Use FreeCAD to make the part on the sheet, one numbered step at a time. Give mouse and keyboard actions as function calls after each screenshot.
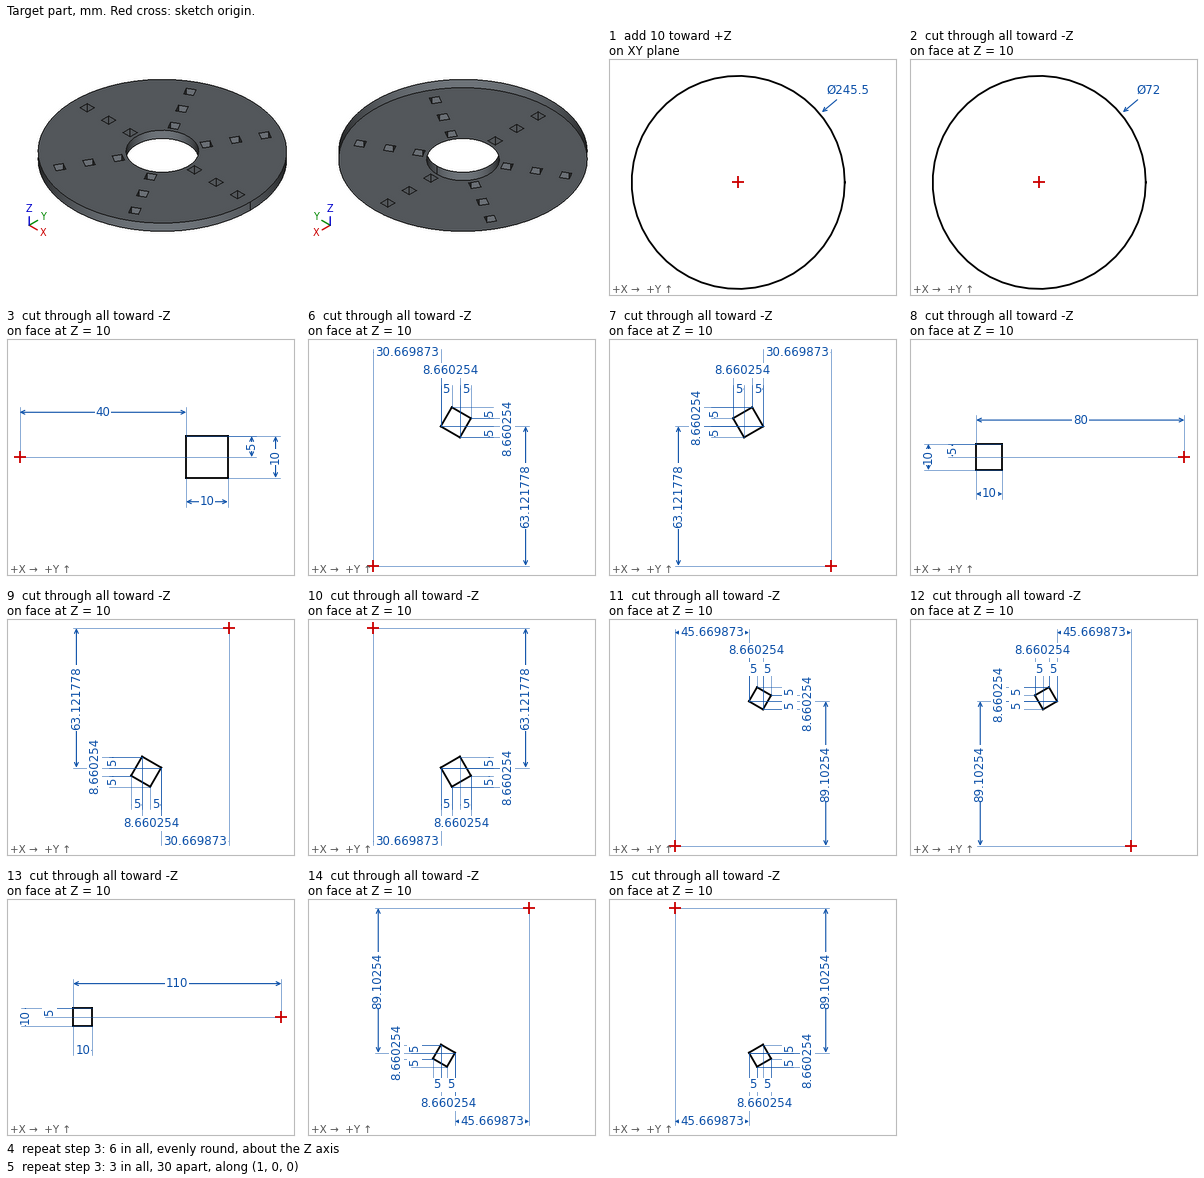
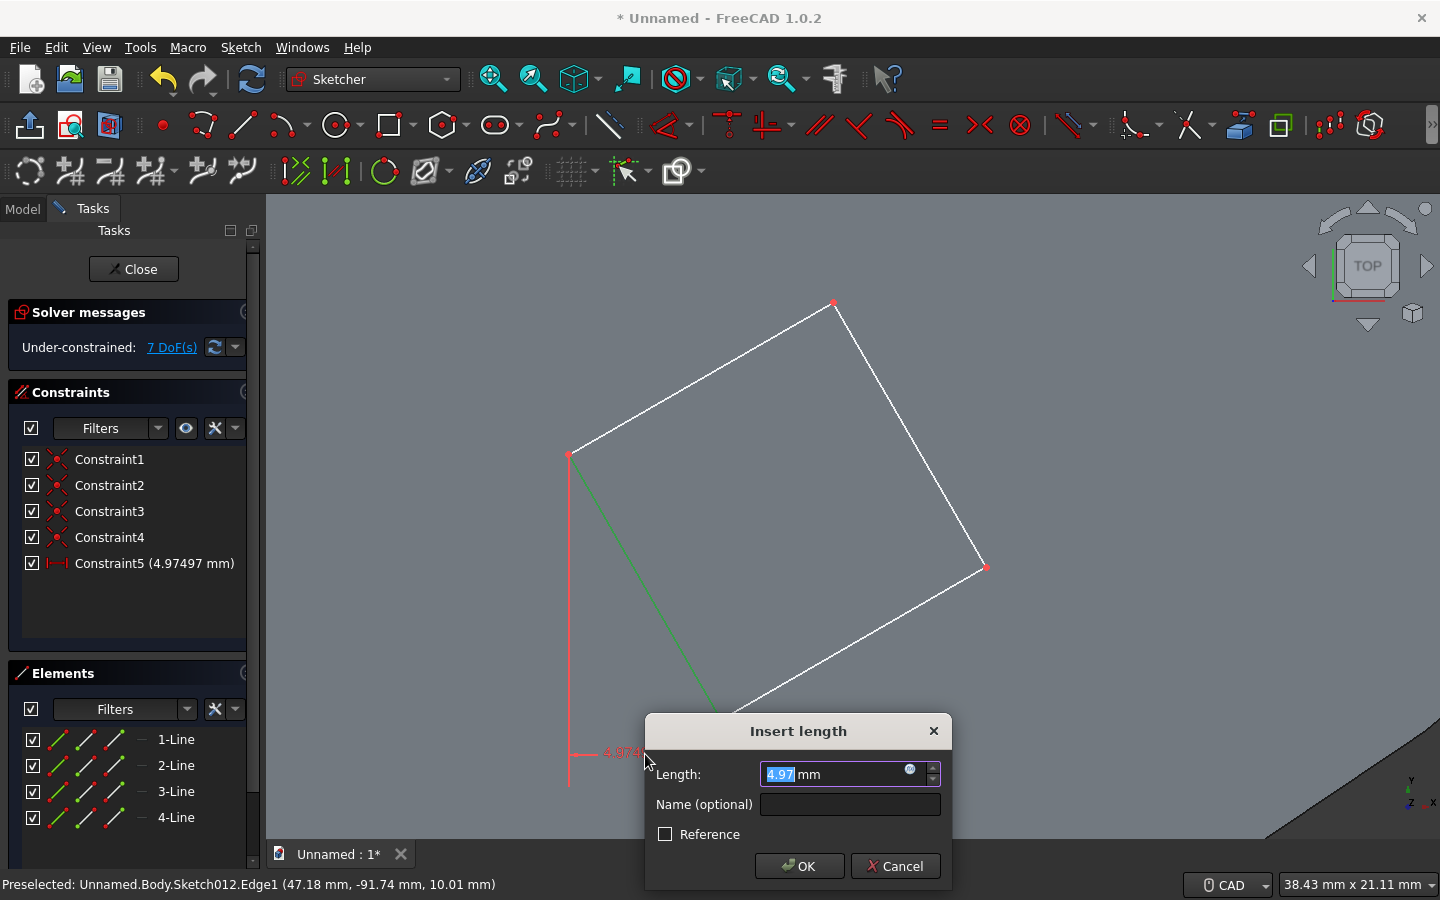
text(5)
key(Return)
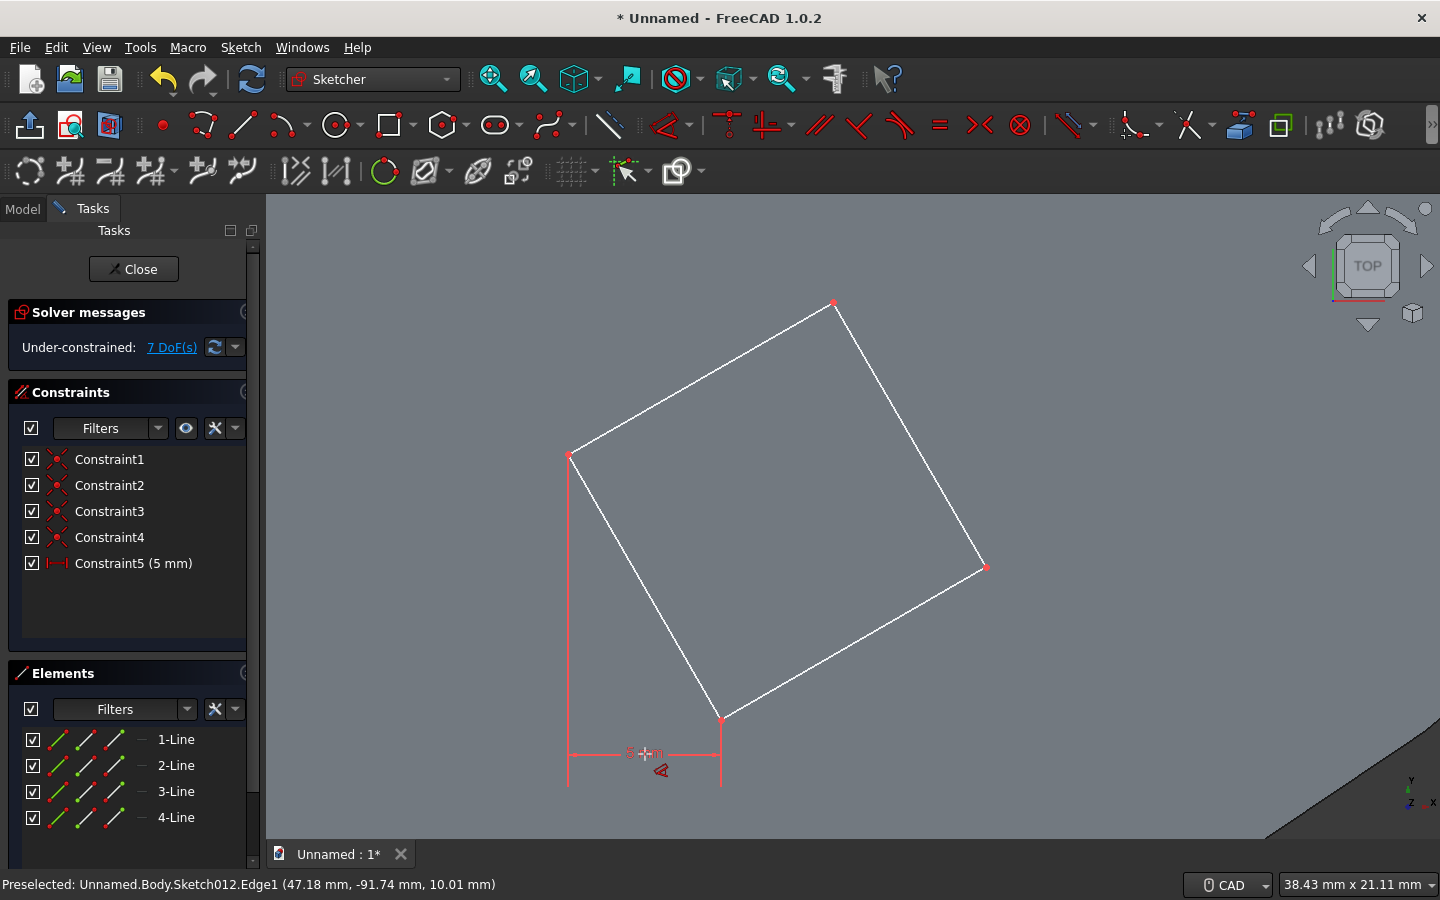
click(801, 674)
click(1020, 644)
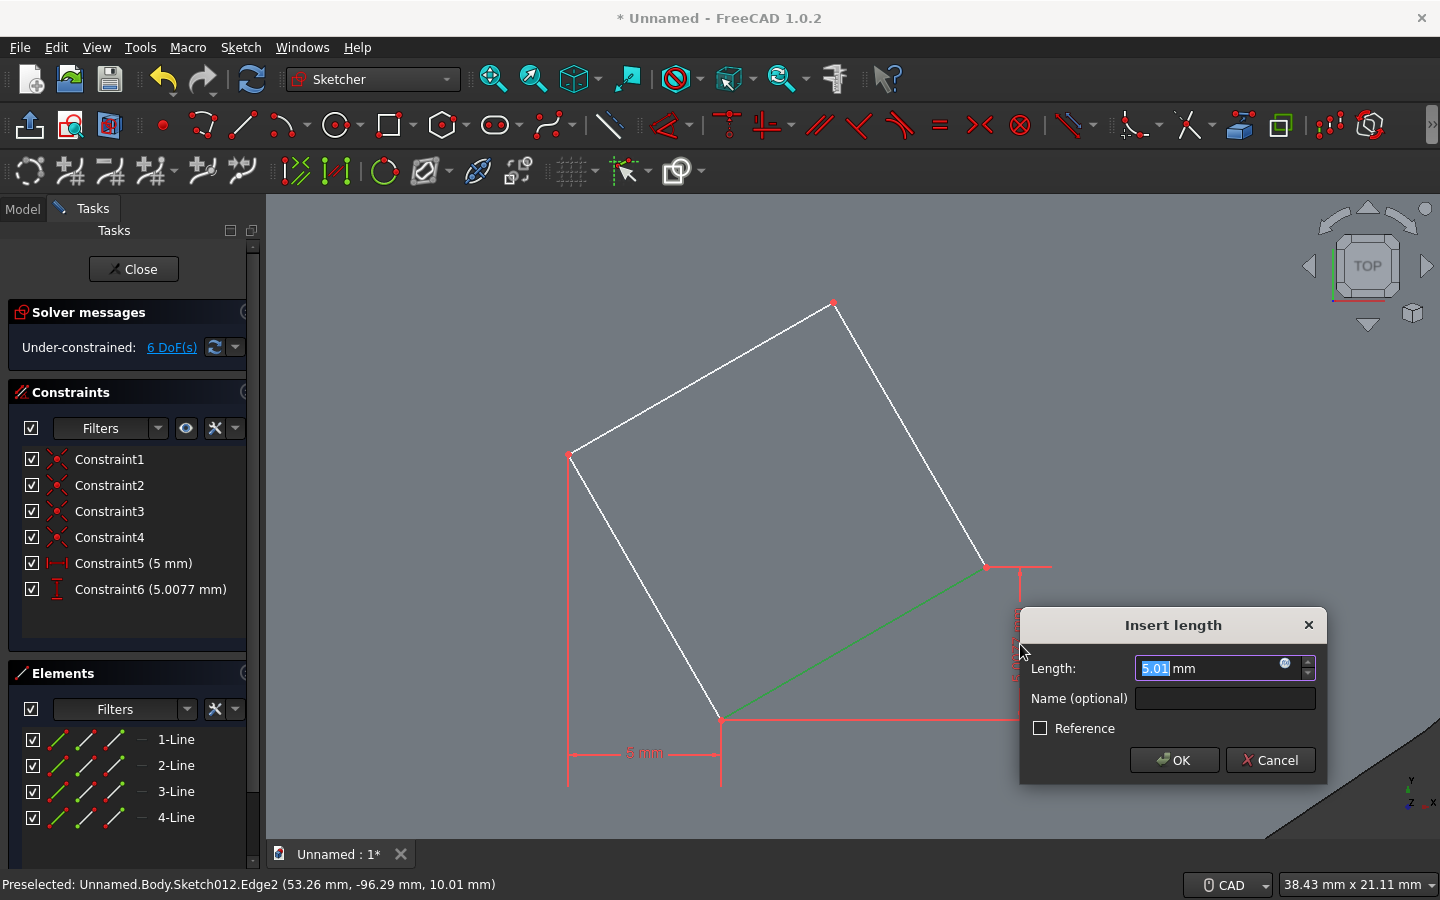
text(5)
key(Return)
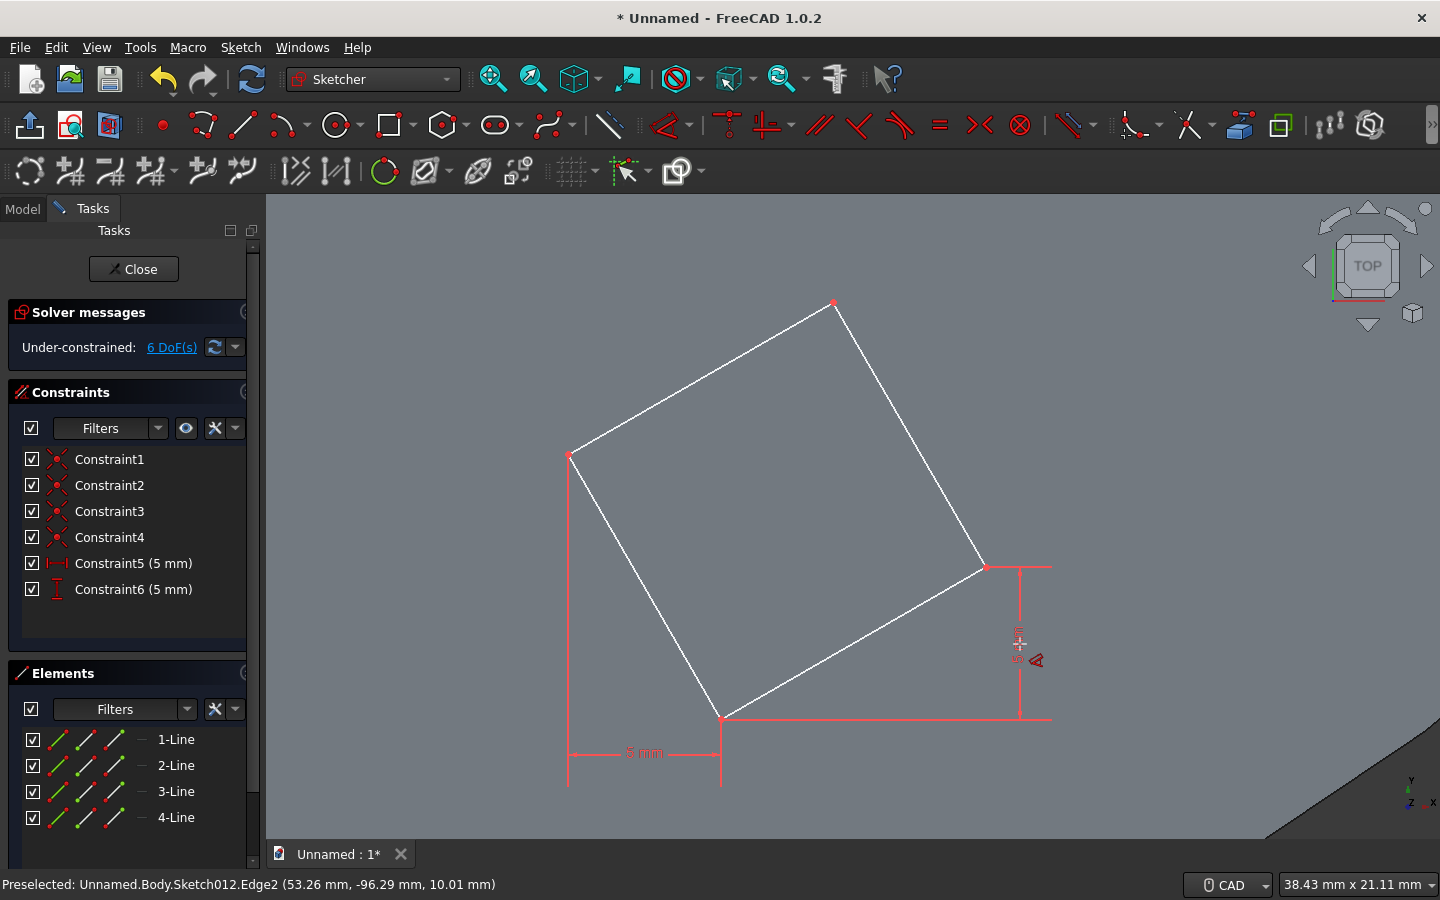
click(940, 488)
click(909, 269)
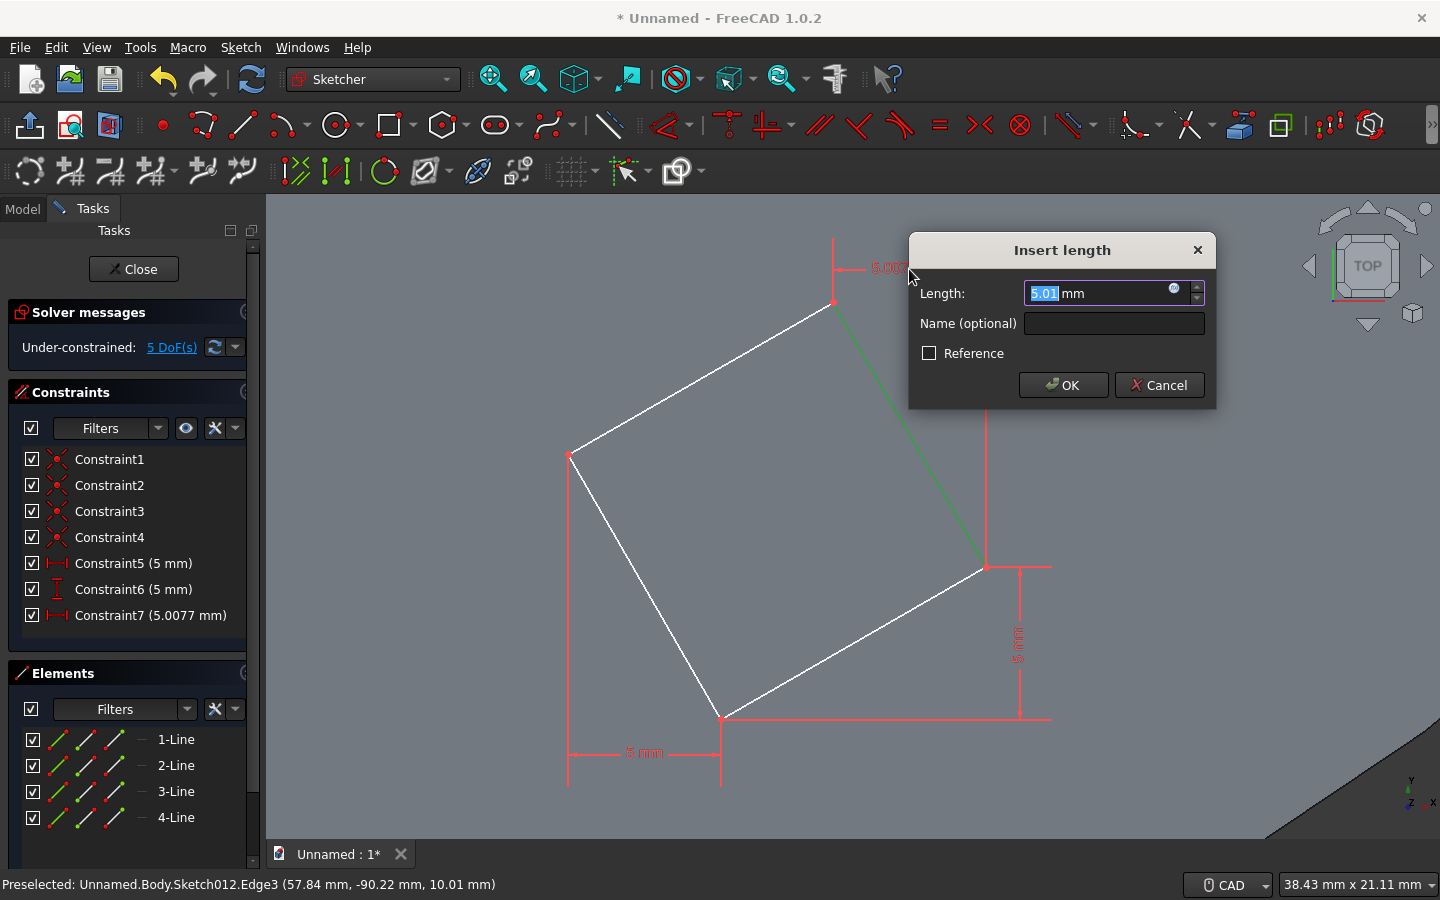
text(5)
key(Return)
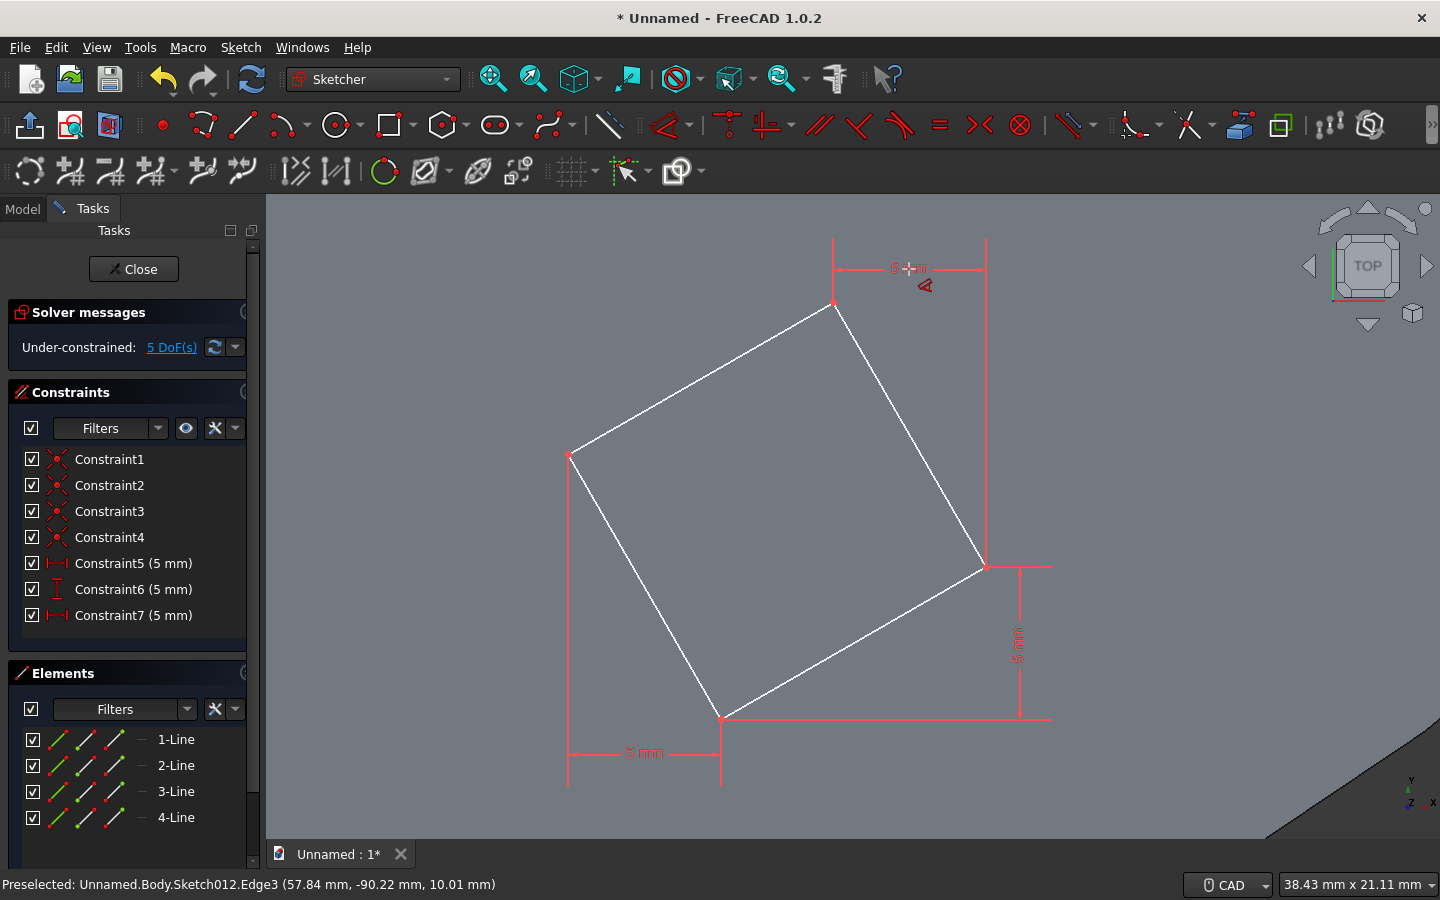
click(754, 349)
click(534, 379)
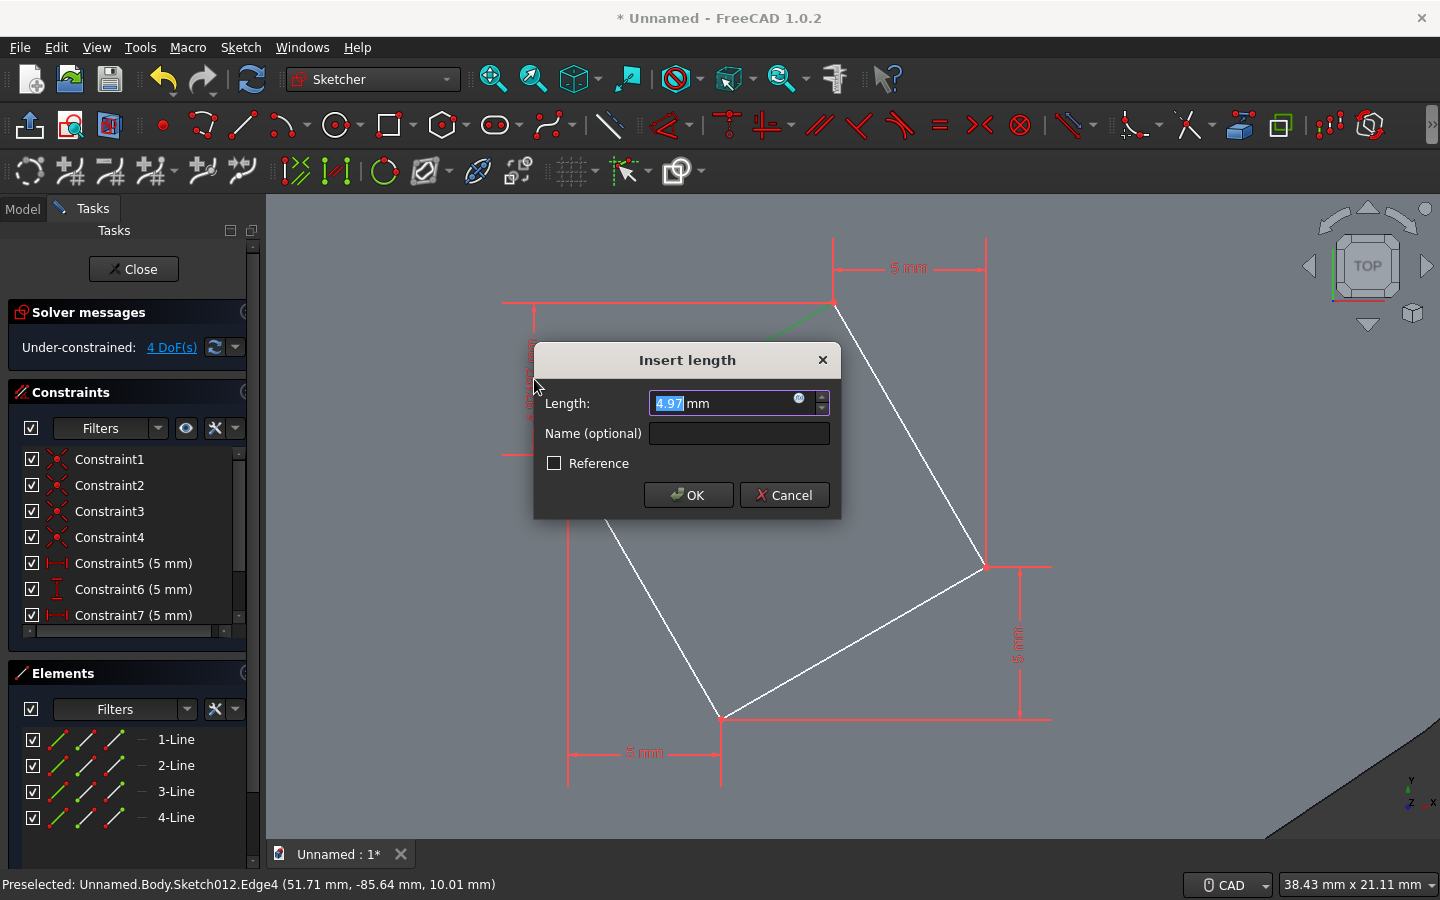
text(5)
key(Return)